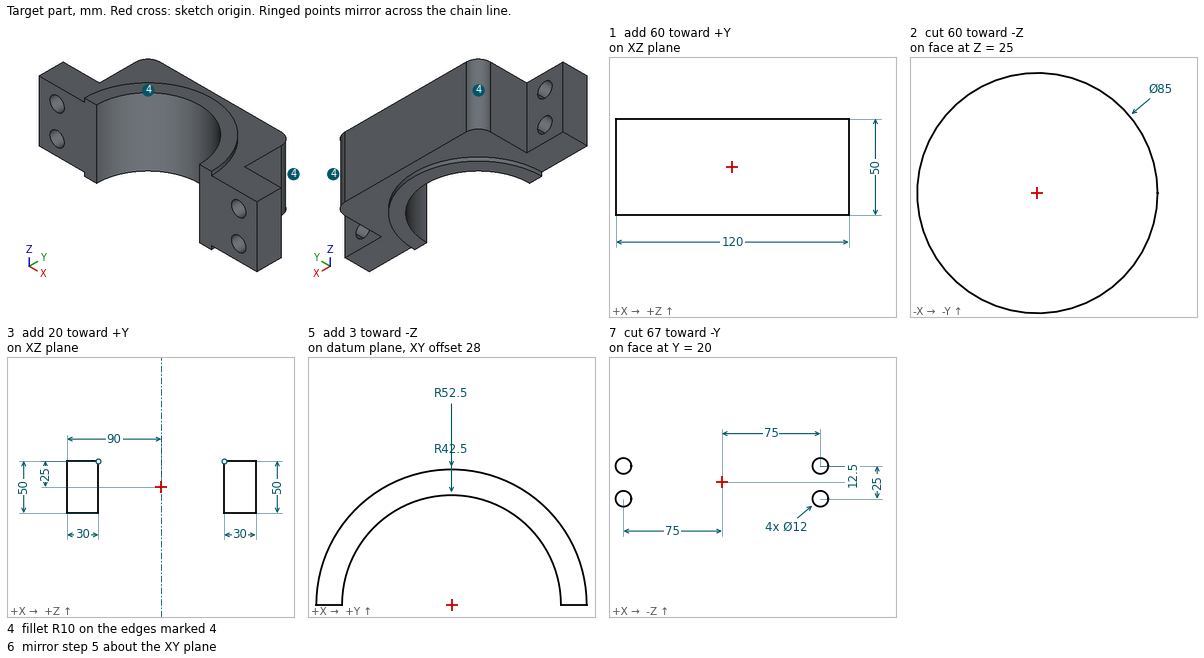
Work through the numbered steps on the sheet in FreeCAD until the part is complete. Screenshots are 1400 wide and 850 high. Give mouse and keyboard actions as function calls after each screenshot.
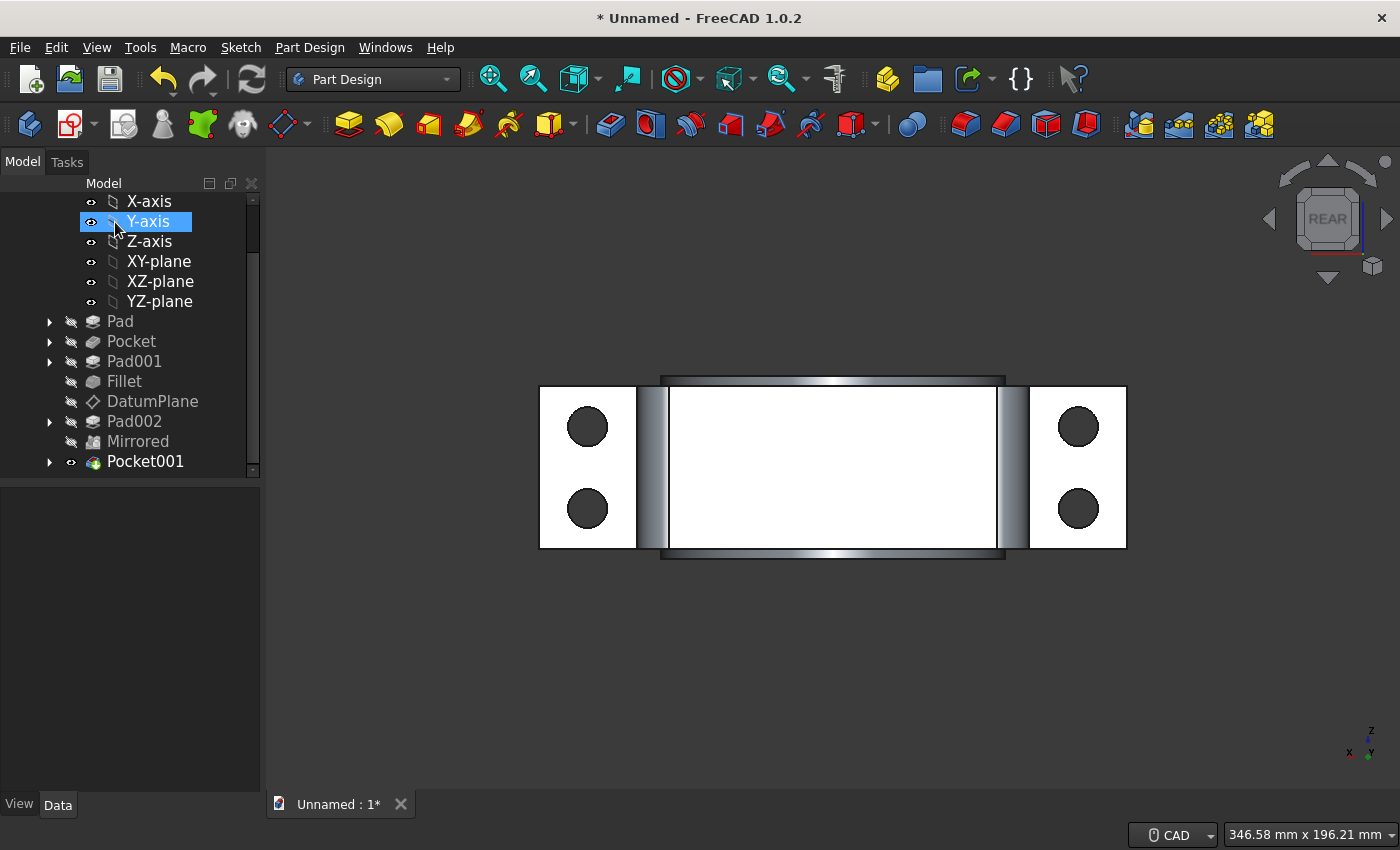
key(0)